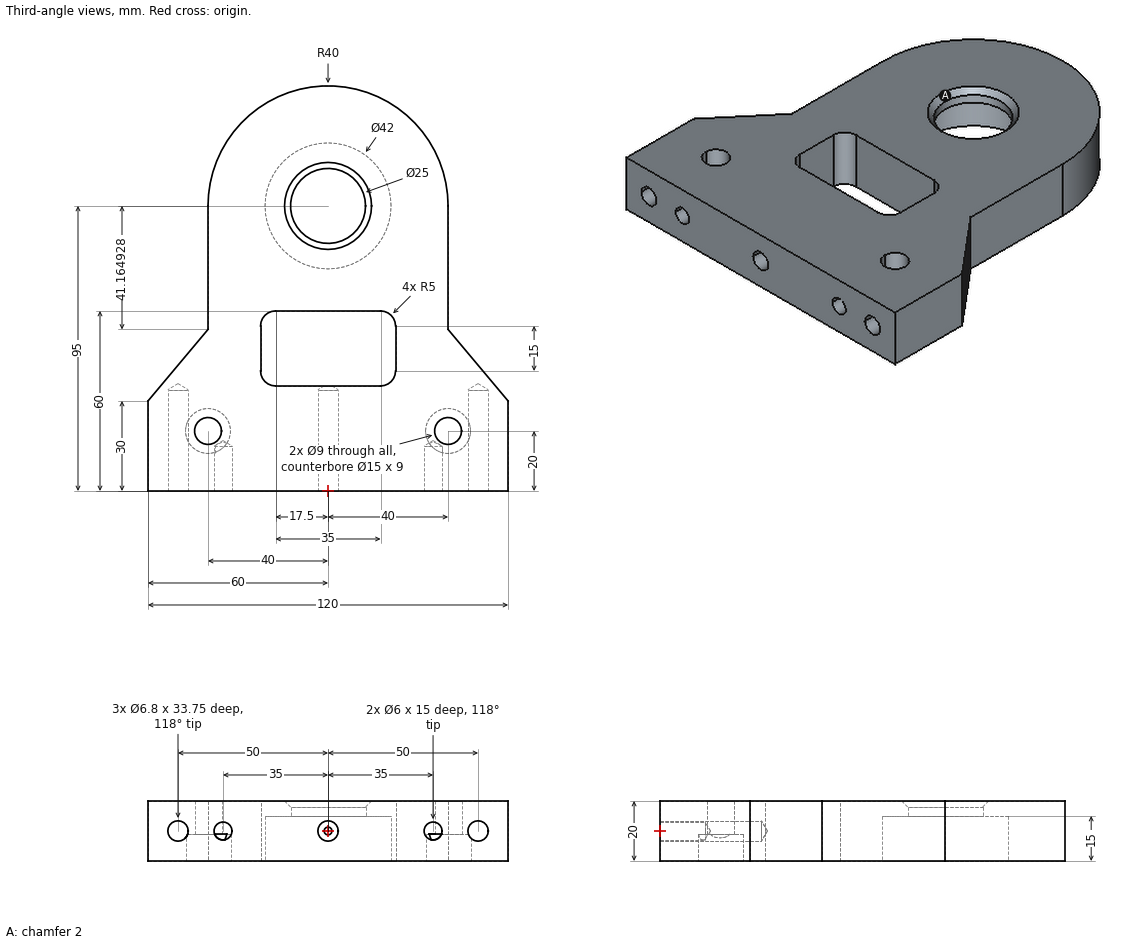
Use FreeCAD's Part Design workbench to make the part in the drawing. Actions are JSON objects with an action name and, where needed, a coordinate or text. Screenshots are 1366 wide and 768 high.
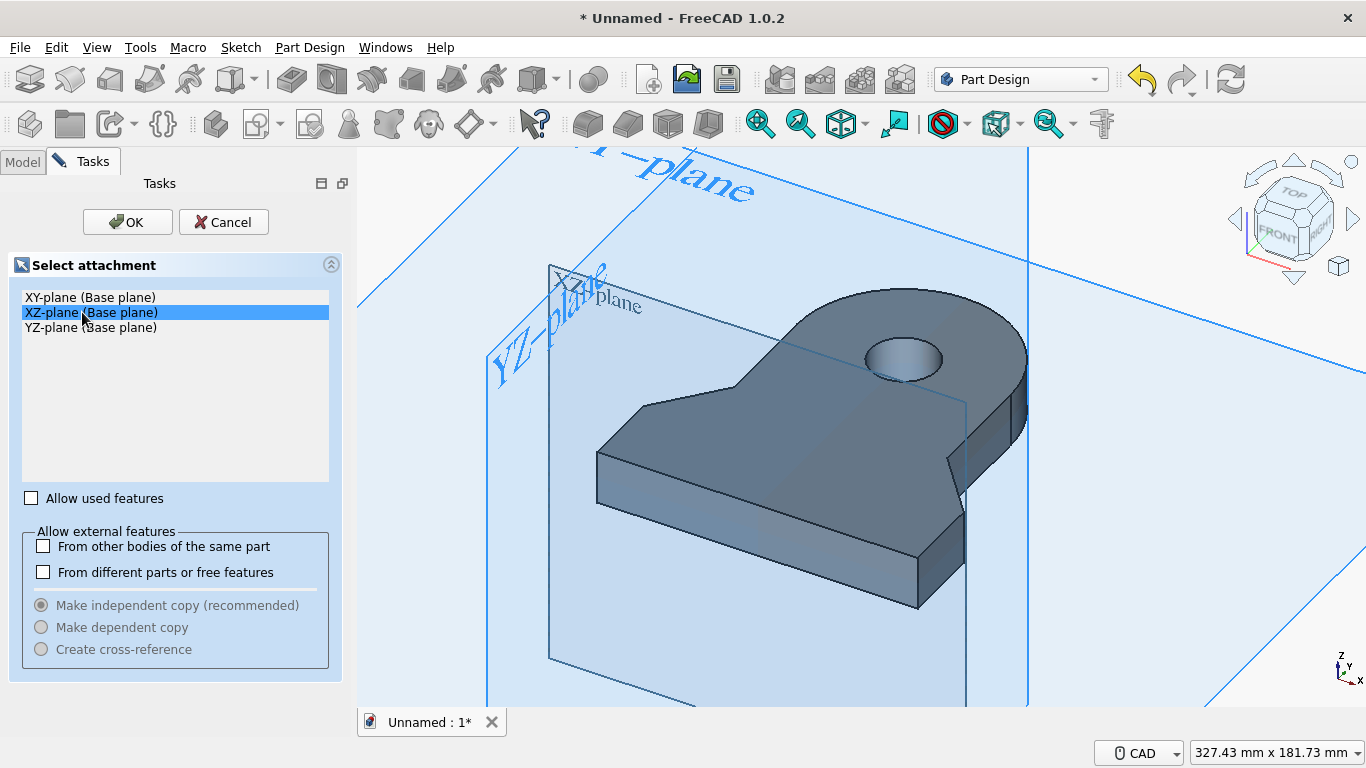
{"action": "left_click", "coordinate": [128, 222]}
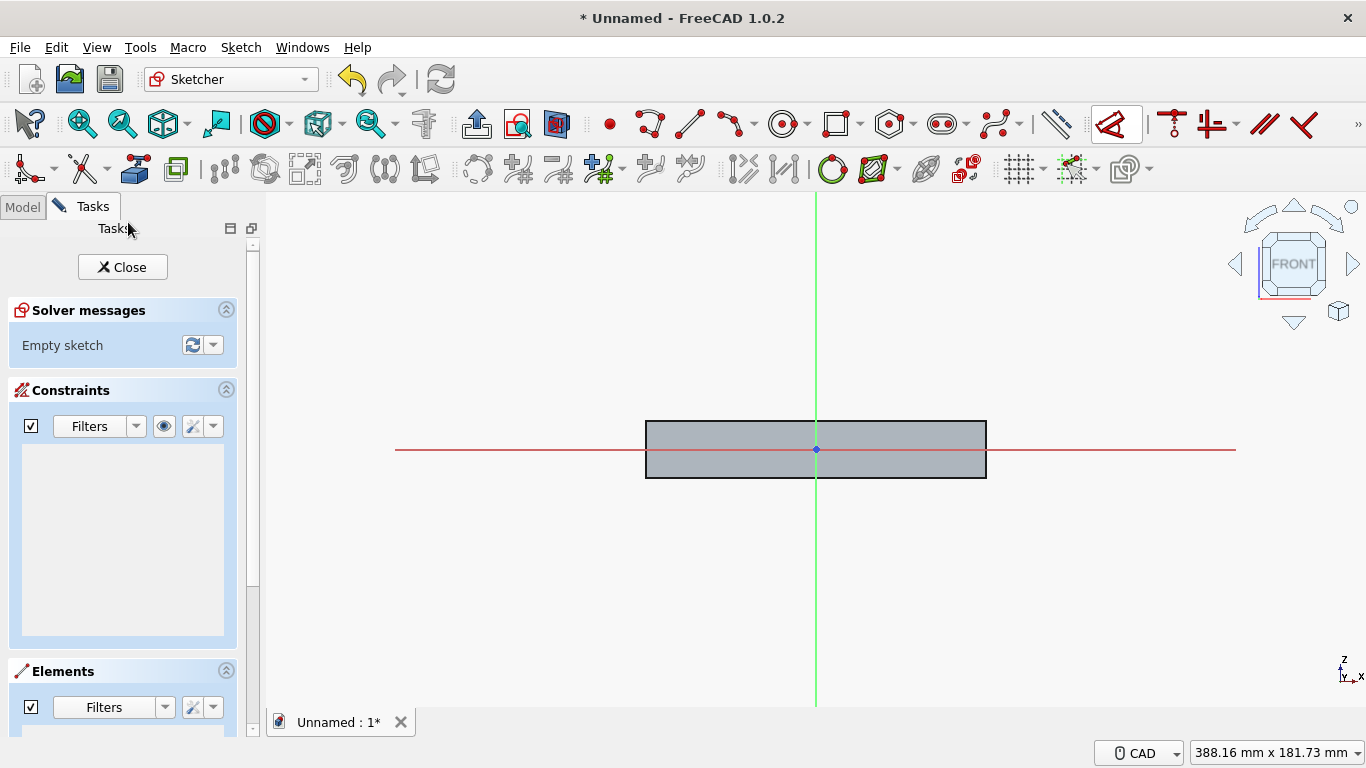
{"action": "scroll", "coordinate": [872, 450], "scroll_direction": "up", "scroll_amount": 4}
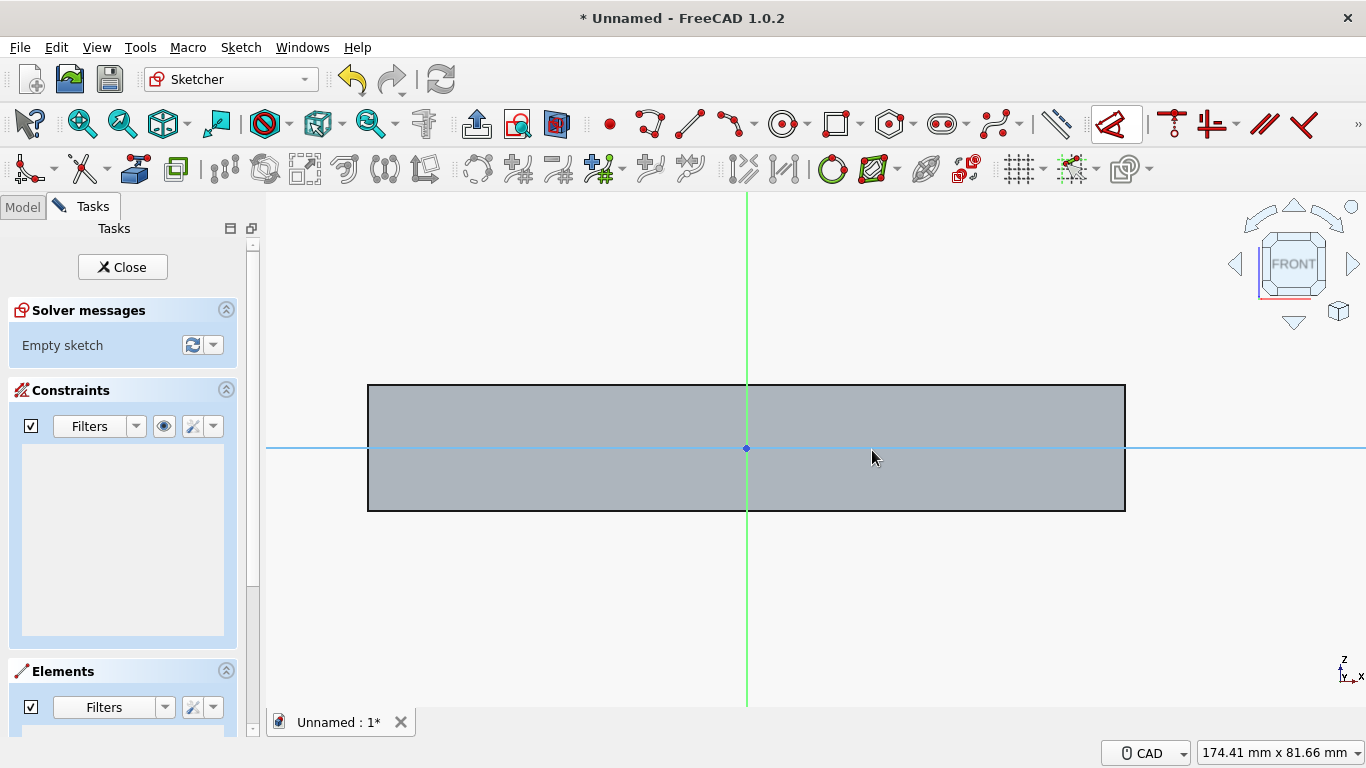
{"action": "left_click", "coordinate": [784, 124]}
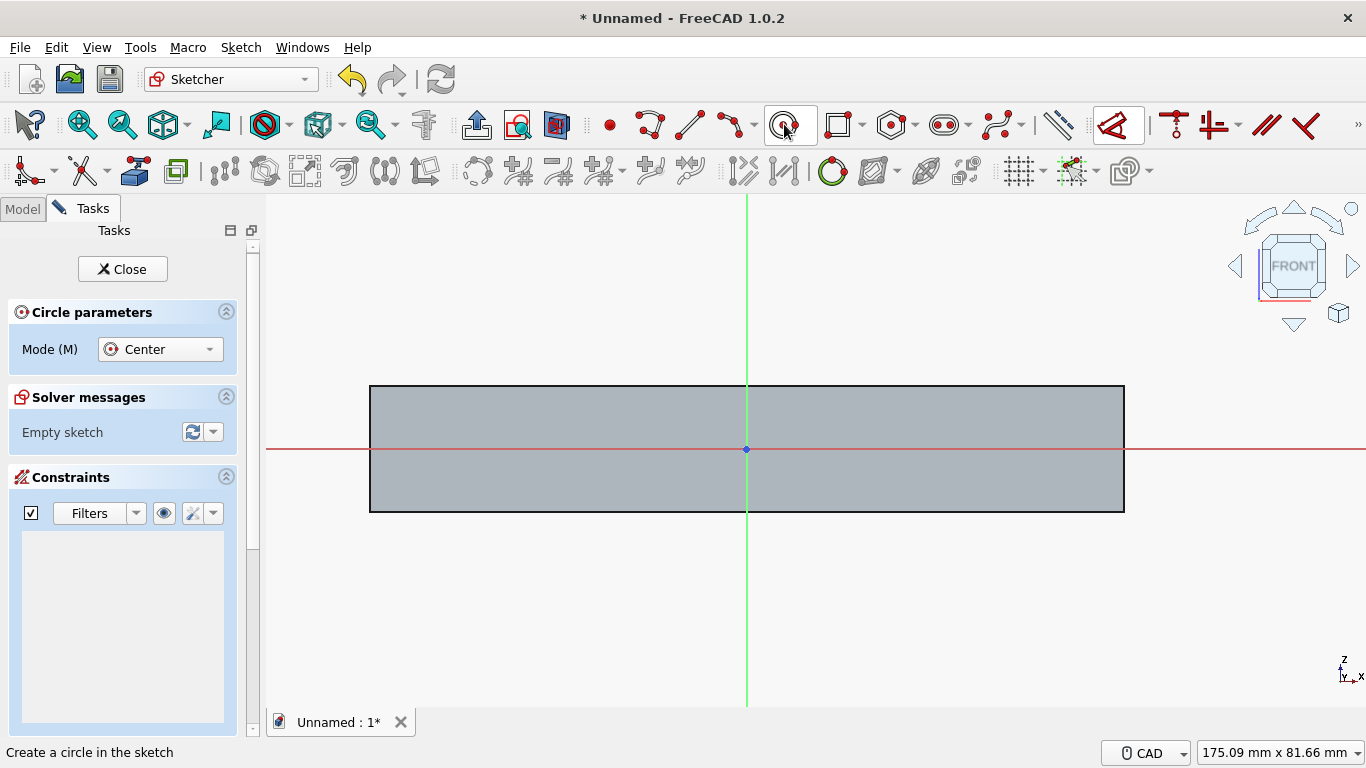
{"action": "left_click", "coordinate": [433, 449]}
{"action": "left_click", "coordinate": [448, 434]}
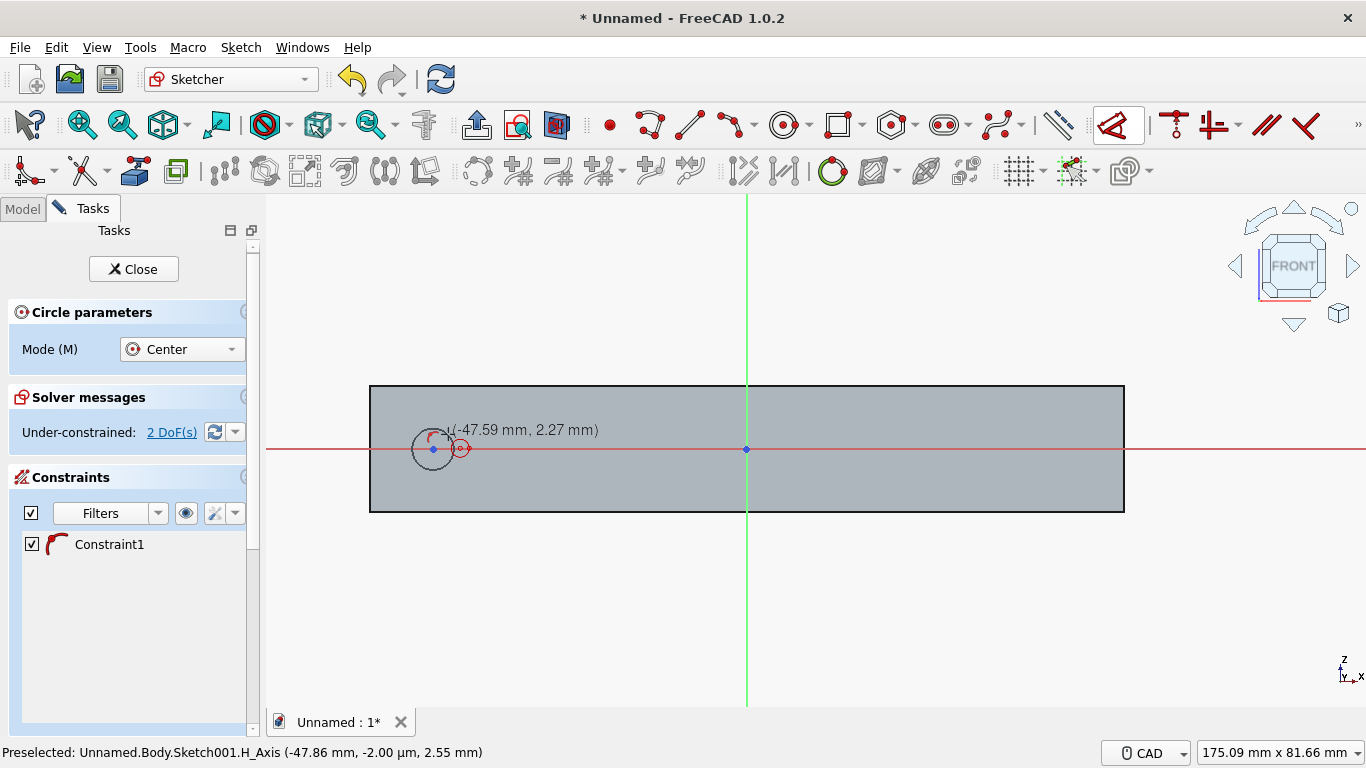
{"action": "left_click", "coordinate": [747, 449]}
{"action": "left_click", "coordinate": [762, 434]}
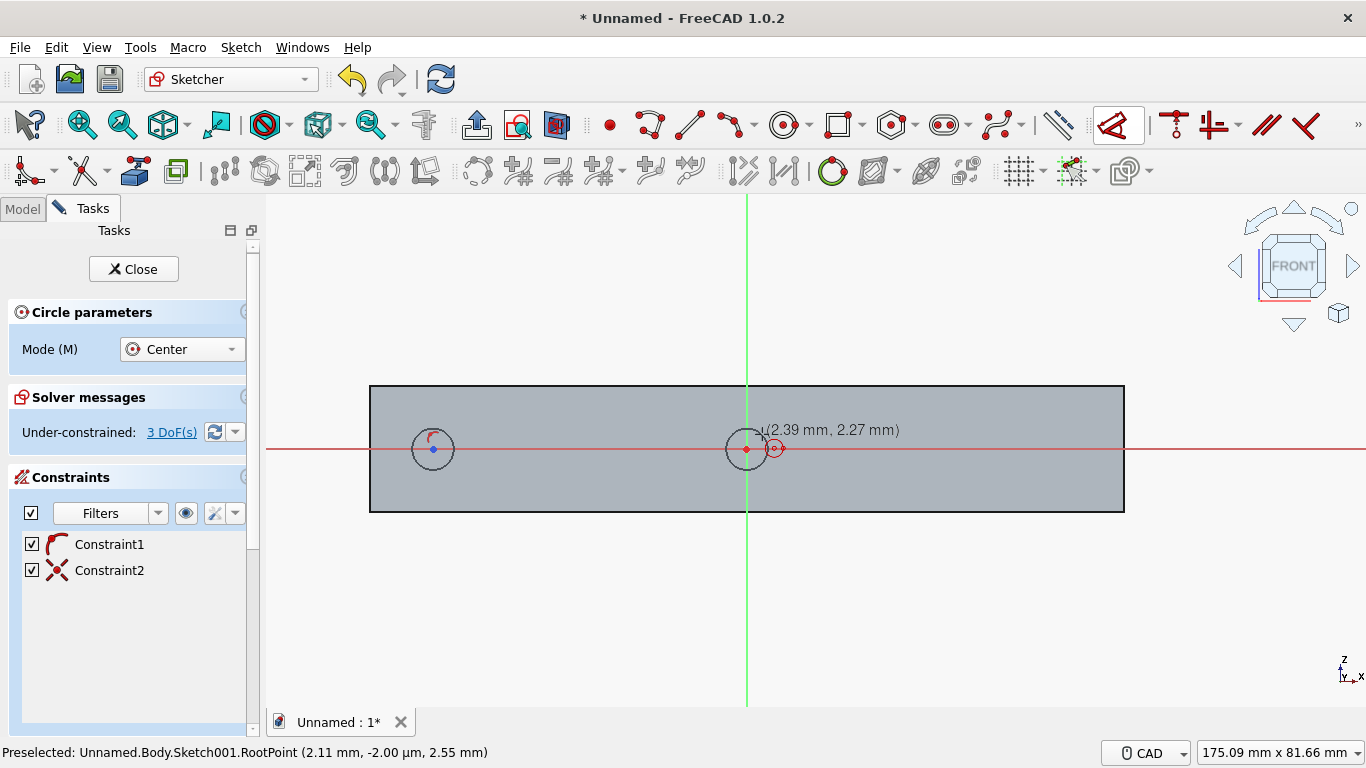
{"action": "left_click", "coordinate": [1061, 449]}
{"action": "left_click", "coordinate": [1076, 434]}
{"action": "key", "text": "Escape"}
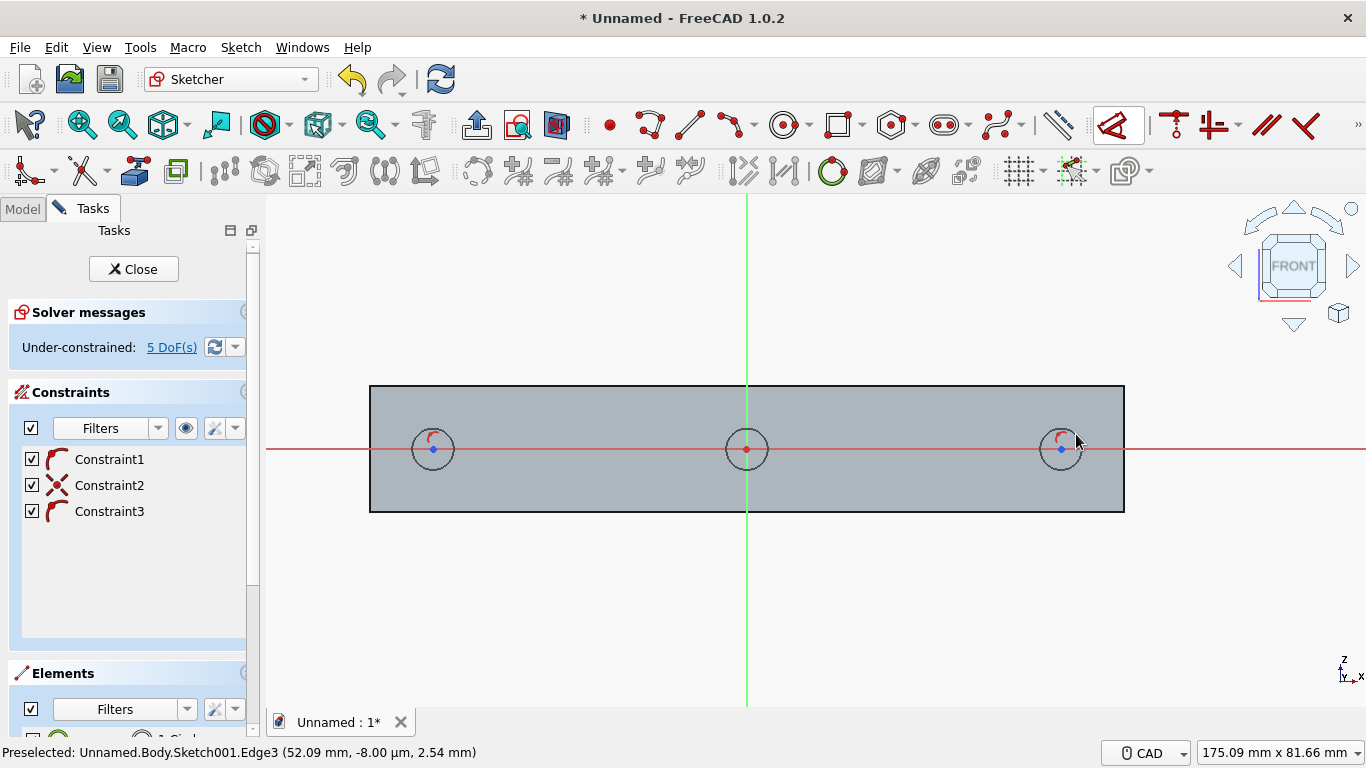
{"action": "left_click", "coordinate": [448, 435]}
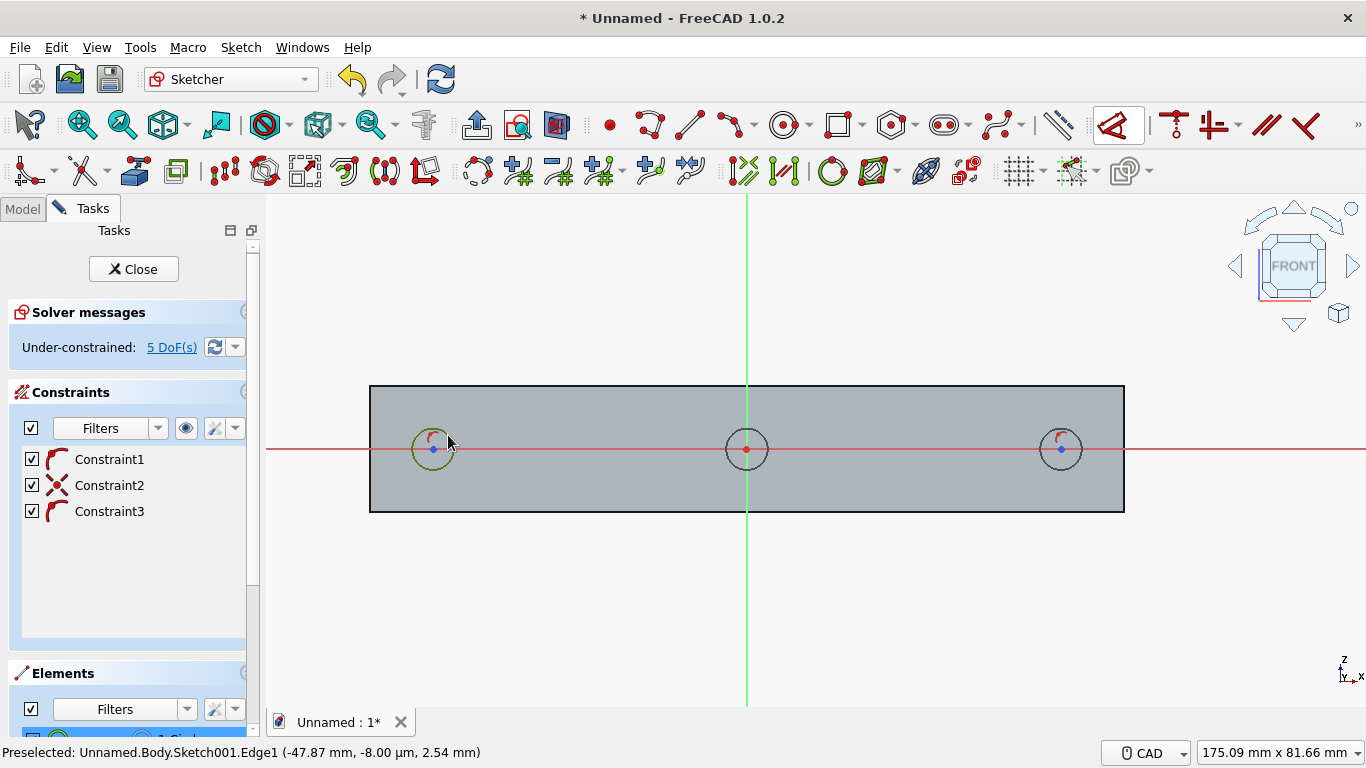
{"action": "left_click", "coordinate": [762, 435]}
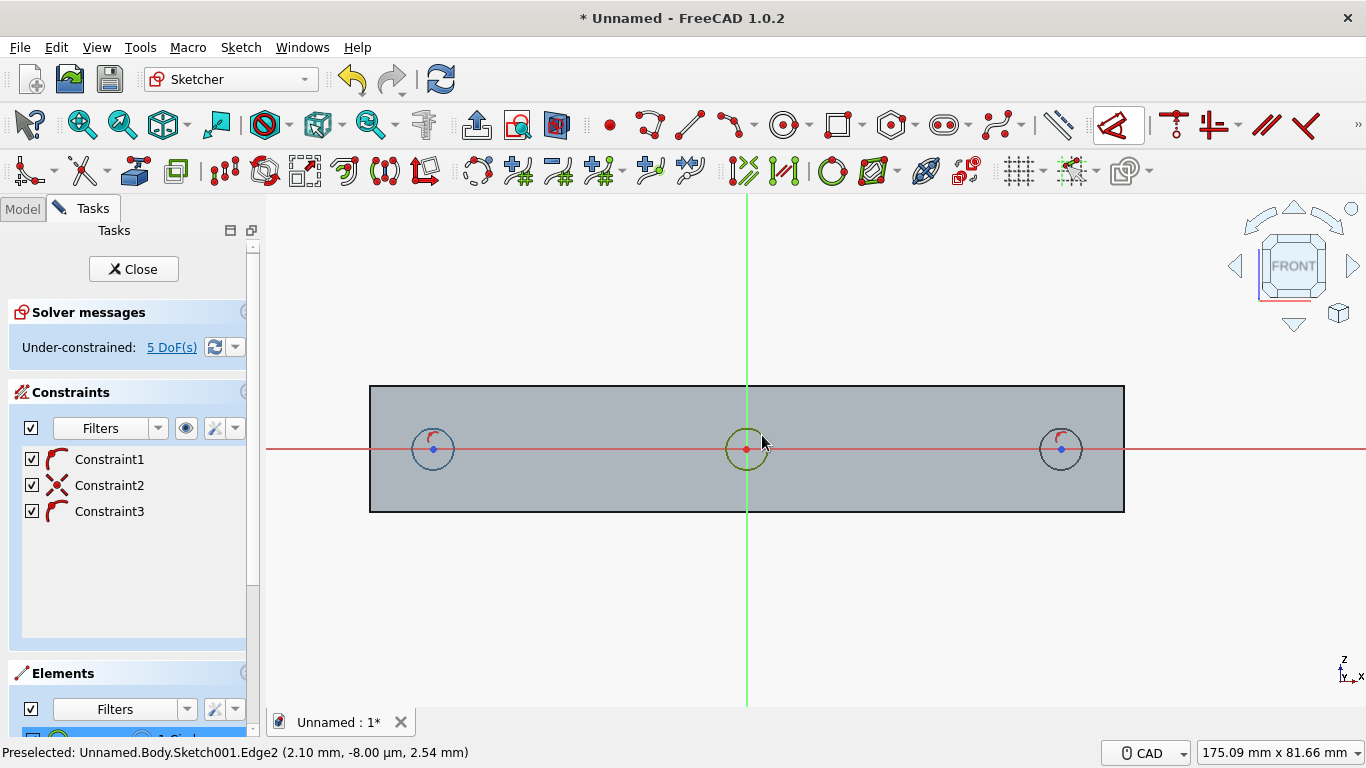
{"action": "left_click", "coordinate": [1076, 435]}